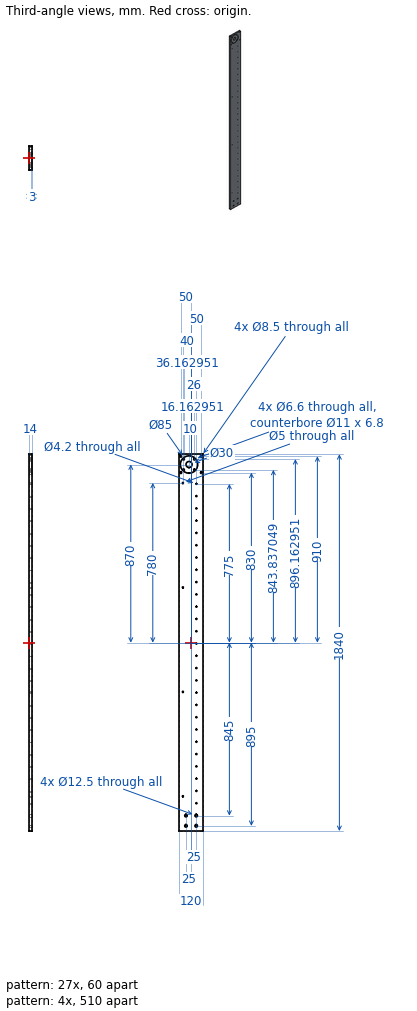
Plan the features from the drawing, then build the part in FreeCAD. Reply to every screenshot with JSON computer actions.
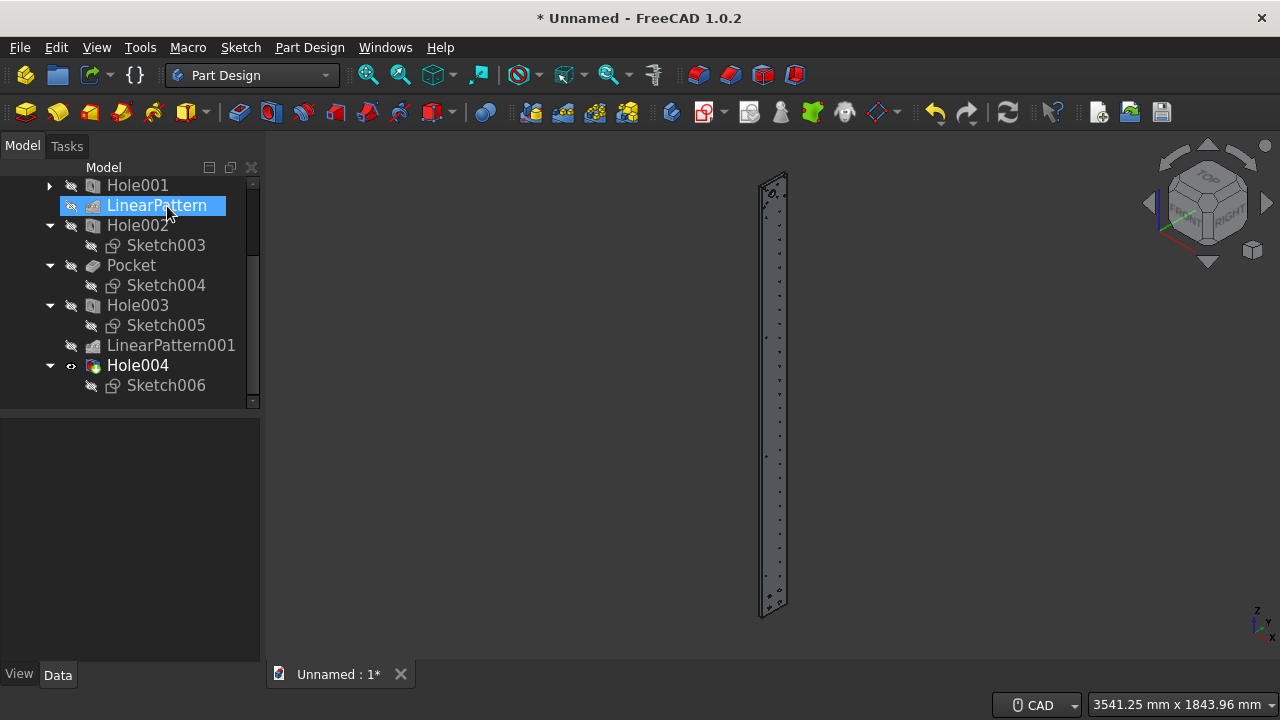
{"action": "left_click", "coordinate": [771, 520]}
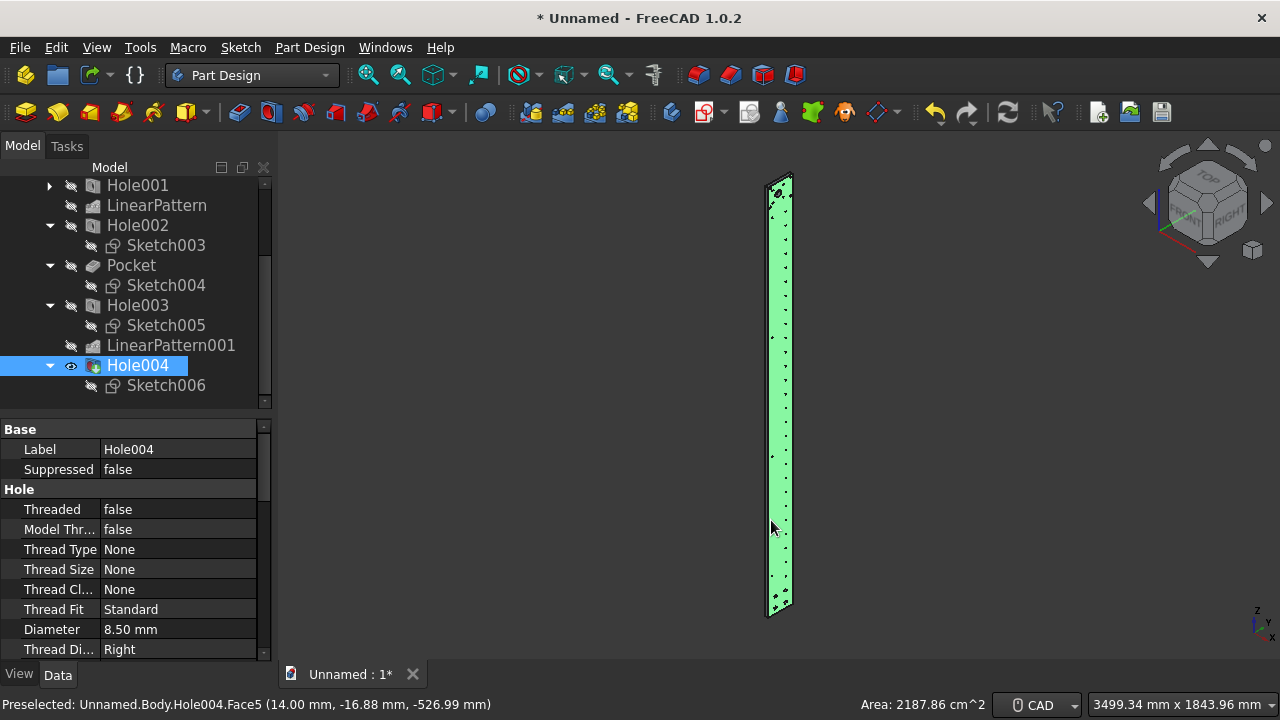
{"action": "left_click", "coordinate": [704, 112]}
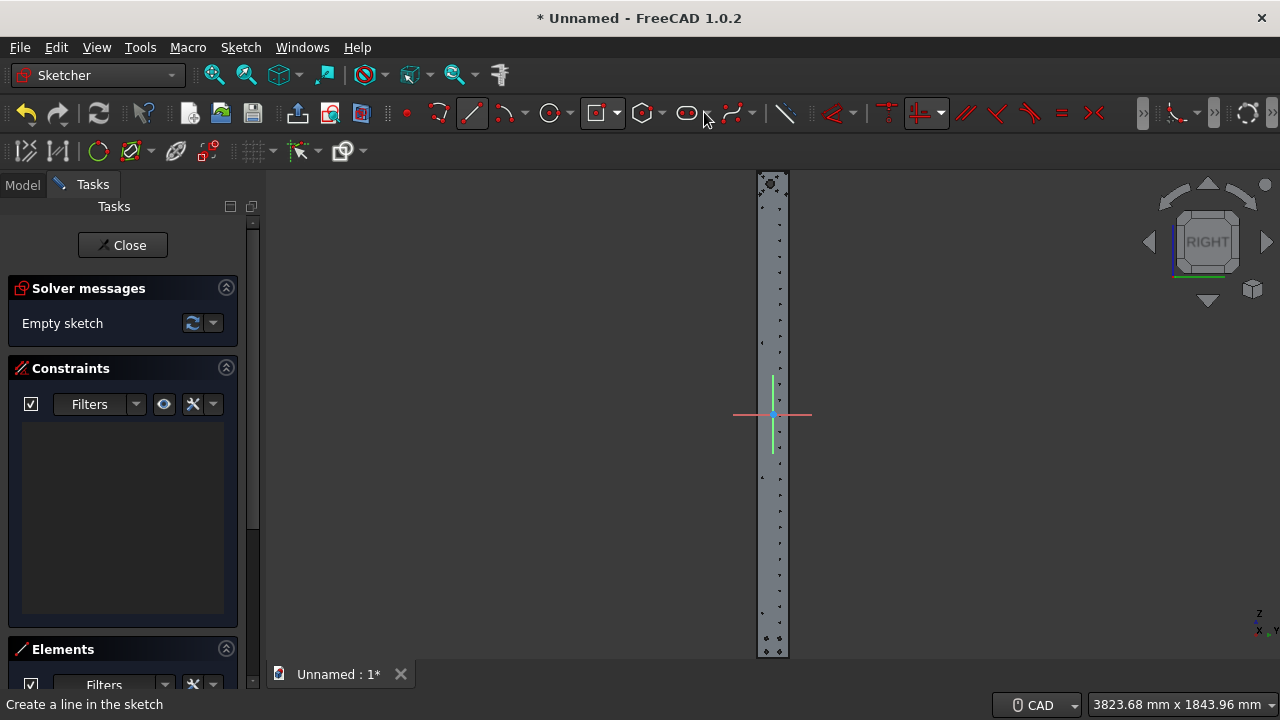
{"action": "scroll", "coordinate": [704, 414], "scroll_direction": "down", "scroll_amount": 5}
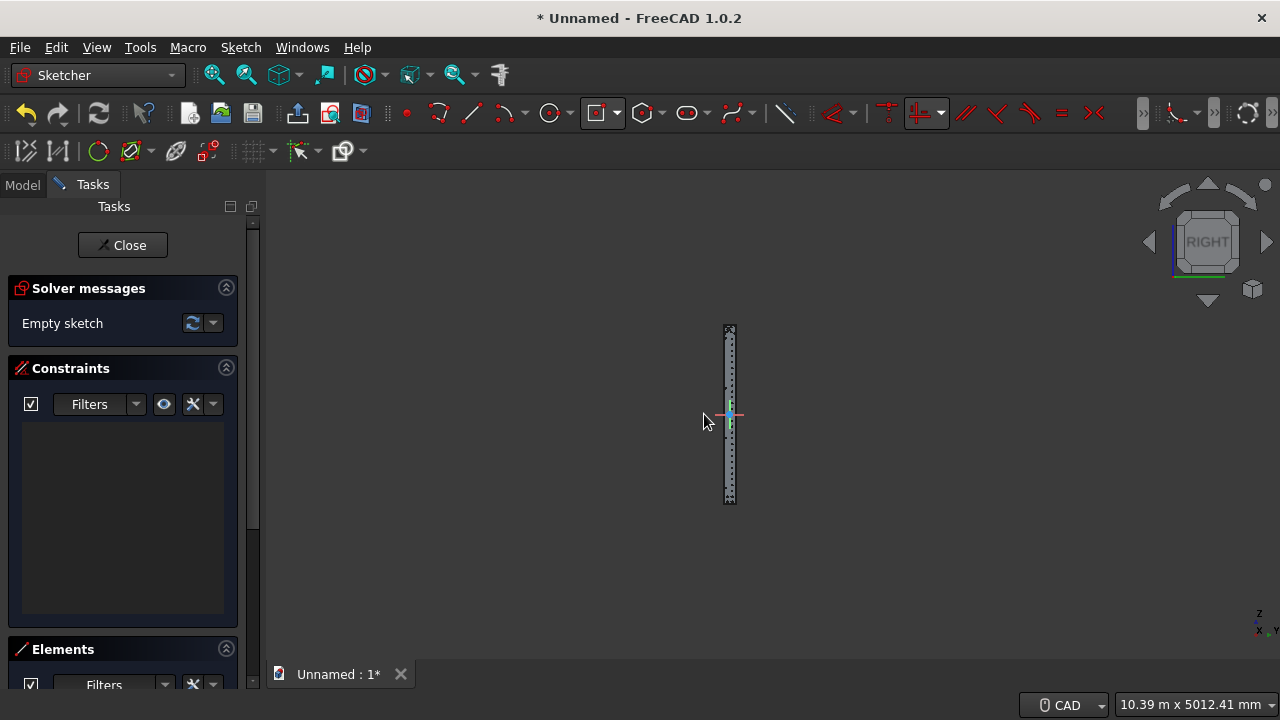
{"action": "scroll", "coordinate": [730, 325], "scroll_direction": "up", "scroll_amount": 15}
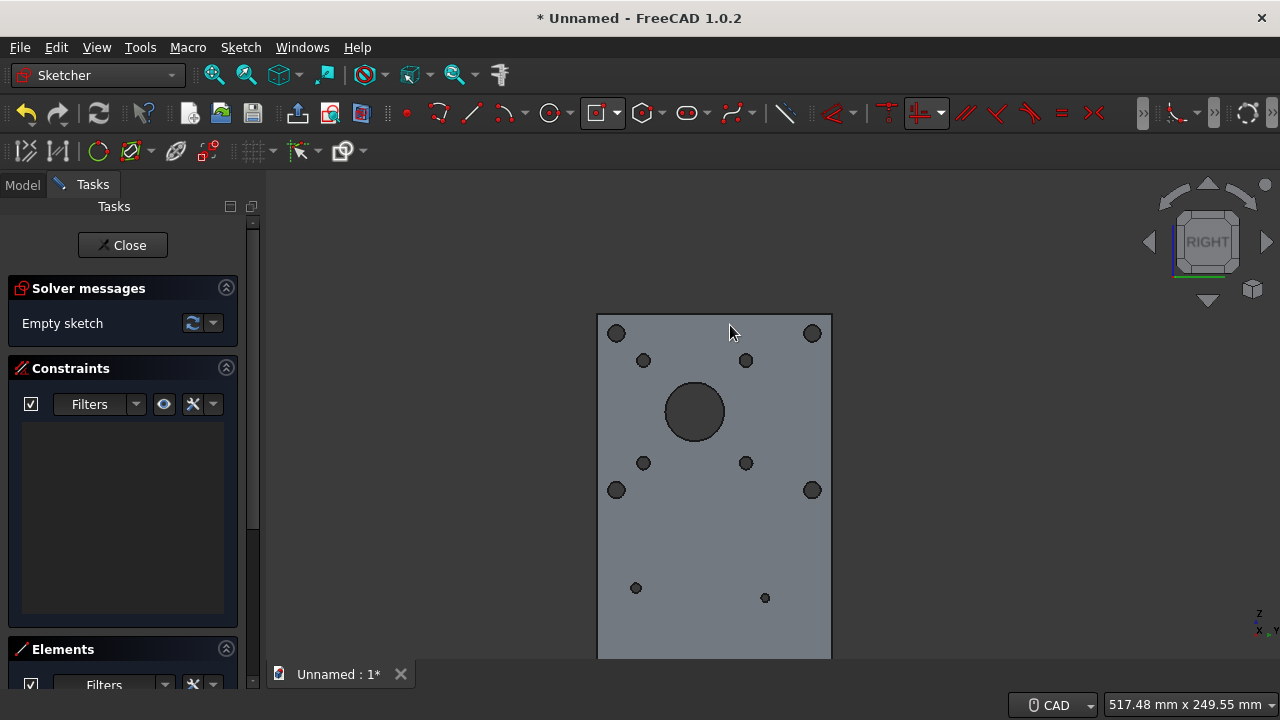
{"action": "scroll", "coordinate": [683, 409], "scroll_direction": "up", "scroll_amount": 3}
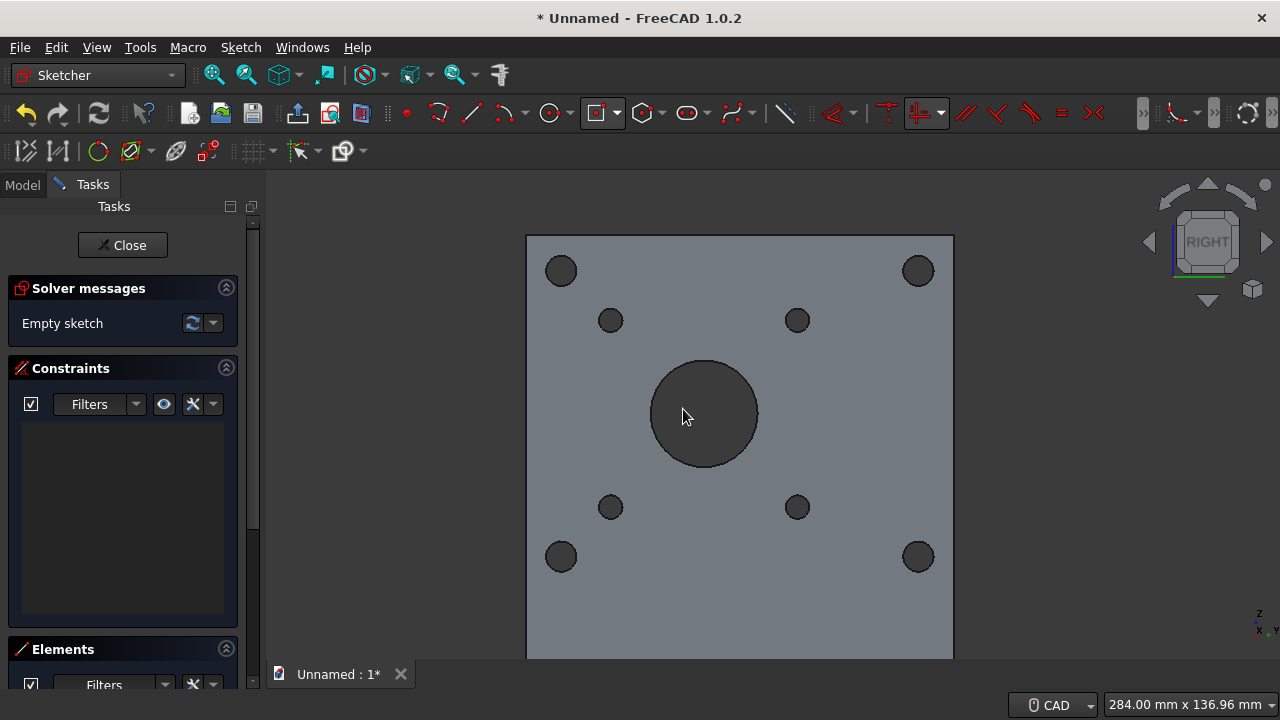
{"action": "left_click", "coordinate": [550, 114]}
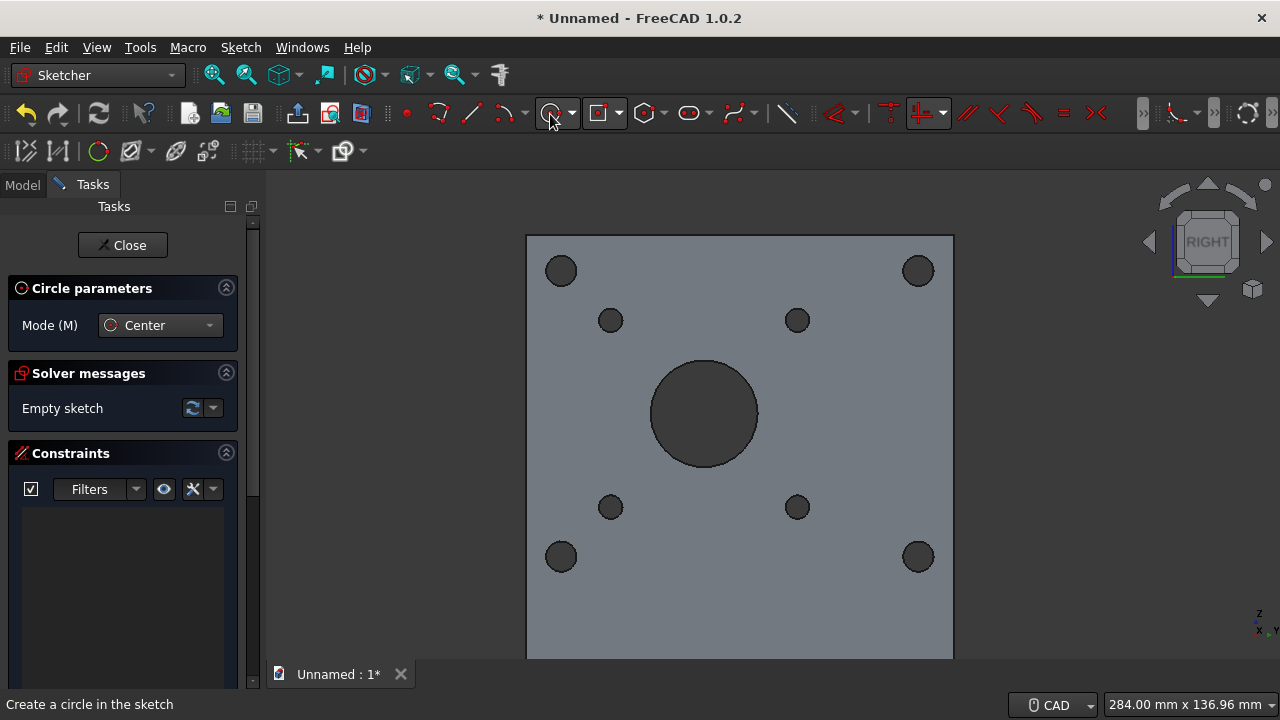
{"action": "left_click", "coordinate": [704, 414]}
{"action": "mouse_move", "coordinate": [811, 306]}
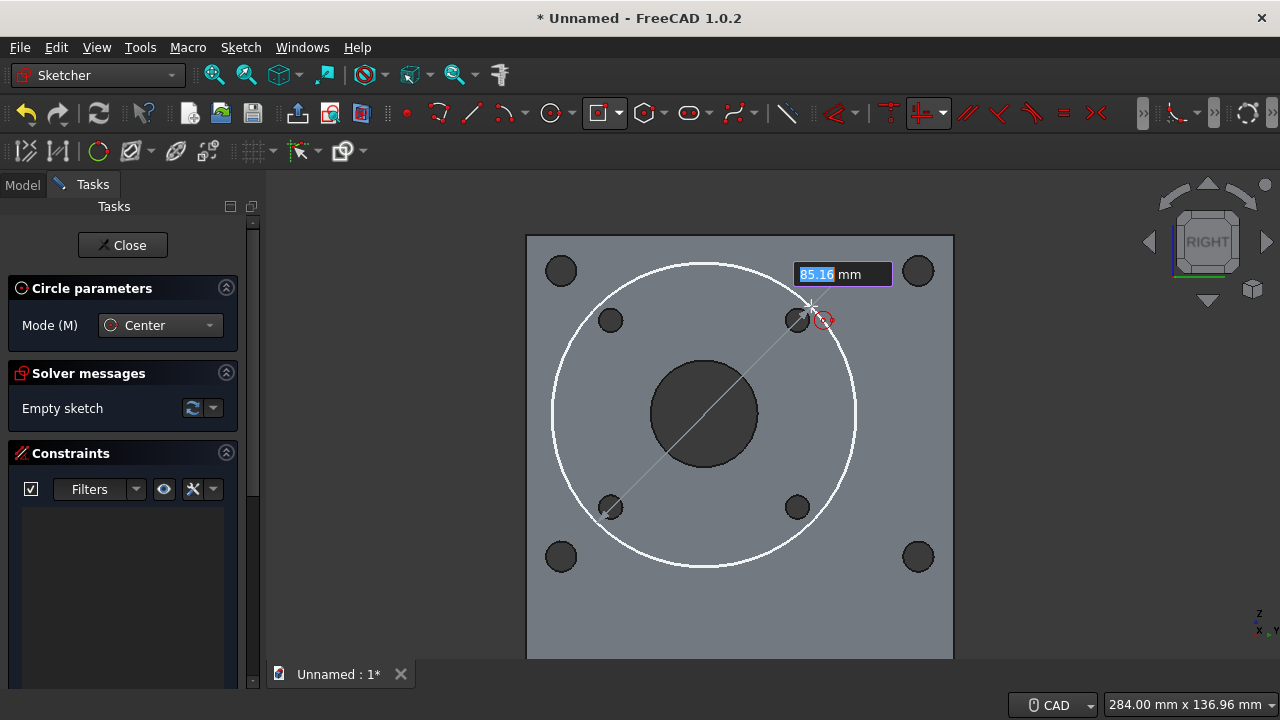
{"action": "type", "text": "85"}
{"action": "key", "text": "Return"}
{"action": "key", "text": "Escape"}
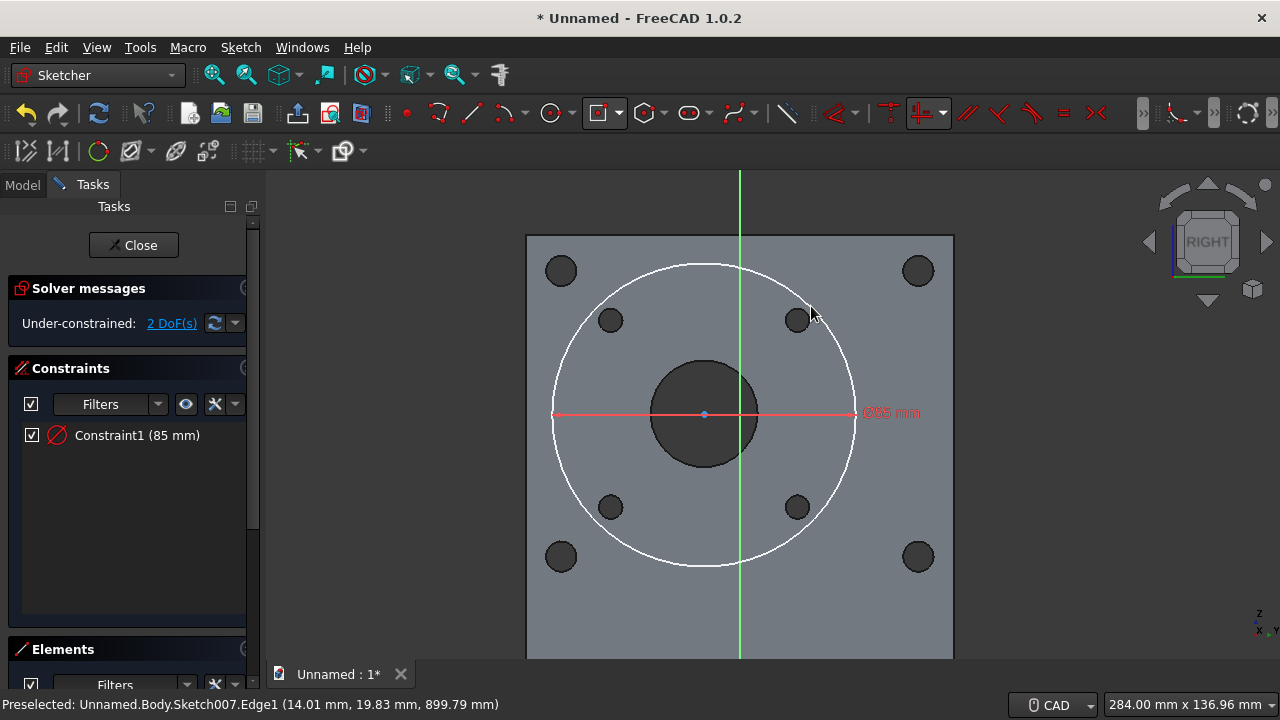
{"action": "left_click", "coordinate": [834, 114]}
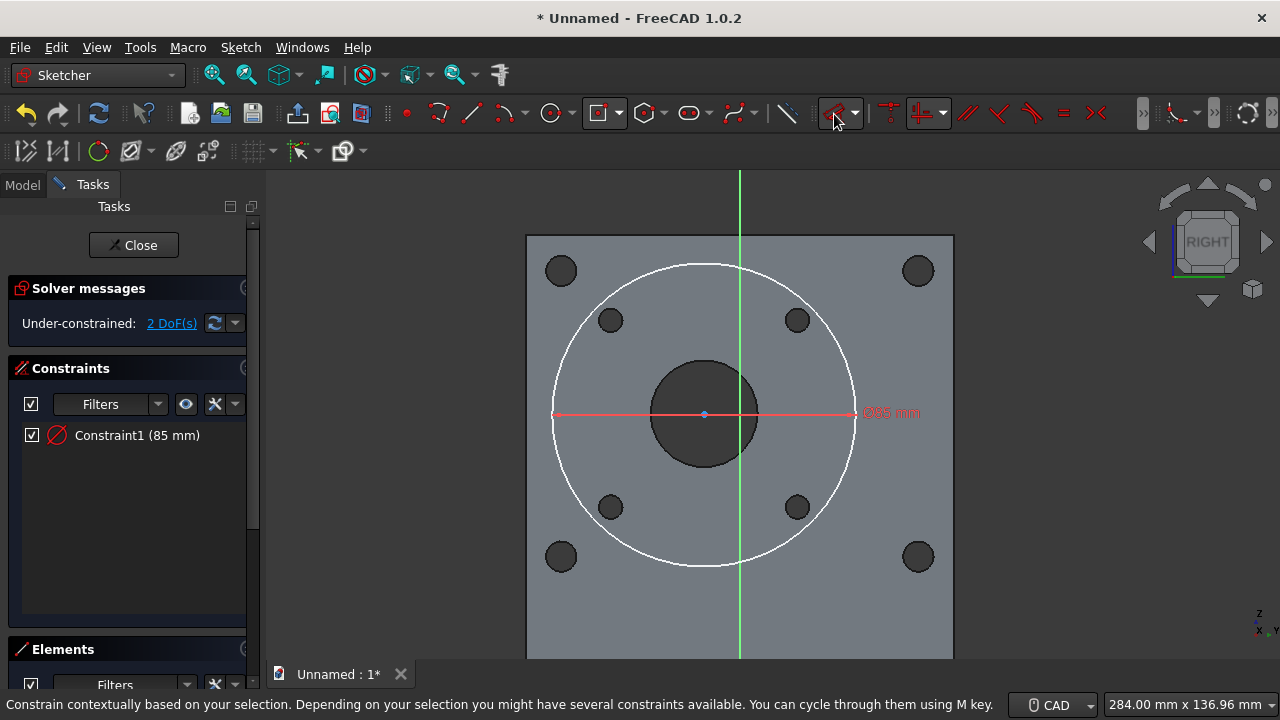
{"action": "left_click", "coordinate": [704, 415]}
{"action": "left_click", "coordinate": [722, 381]}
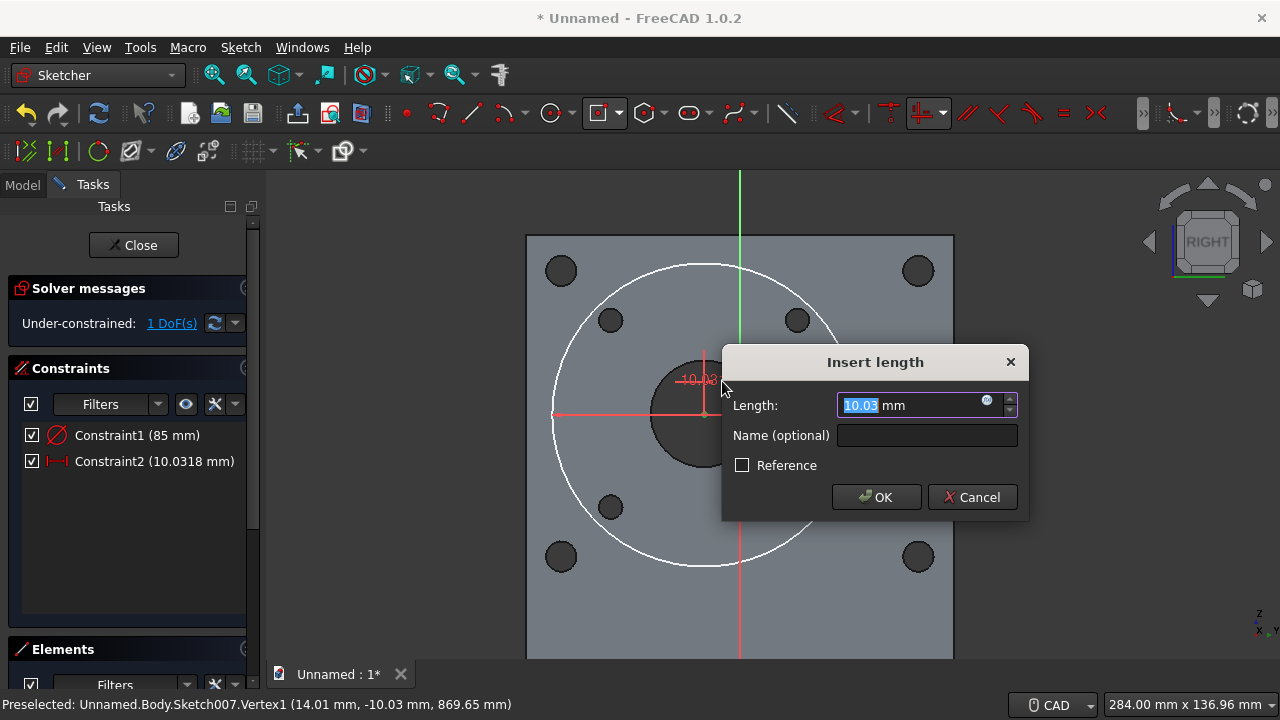
{"action": "type", "text": "10"}
{"action": "key", "text": "Return"}